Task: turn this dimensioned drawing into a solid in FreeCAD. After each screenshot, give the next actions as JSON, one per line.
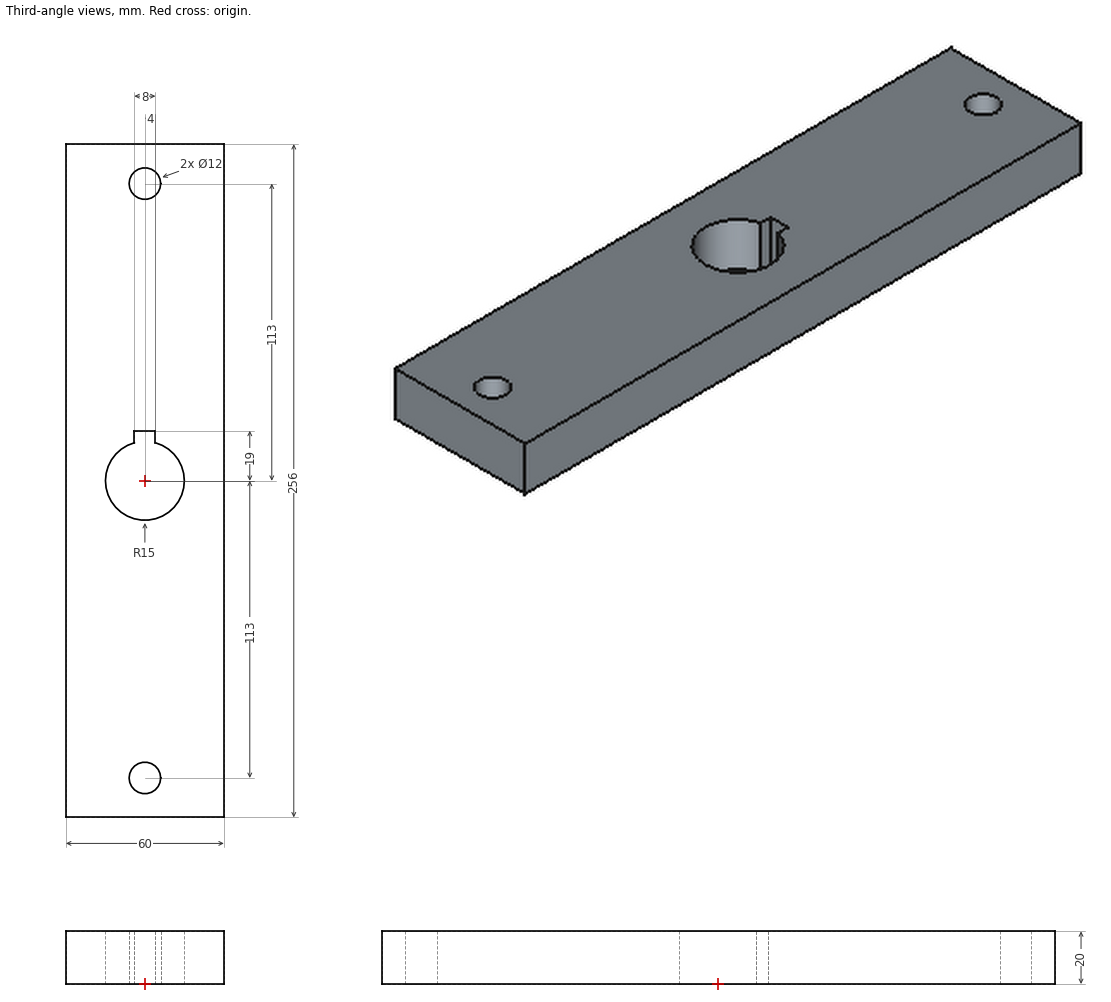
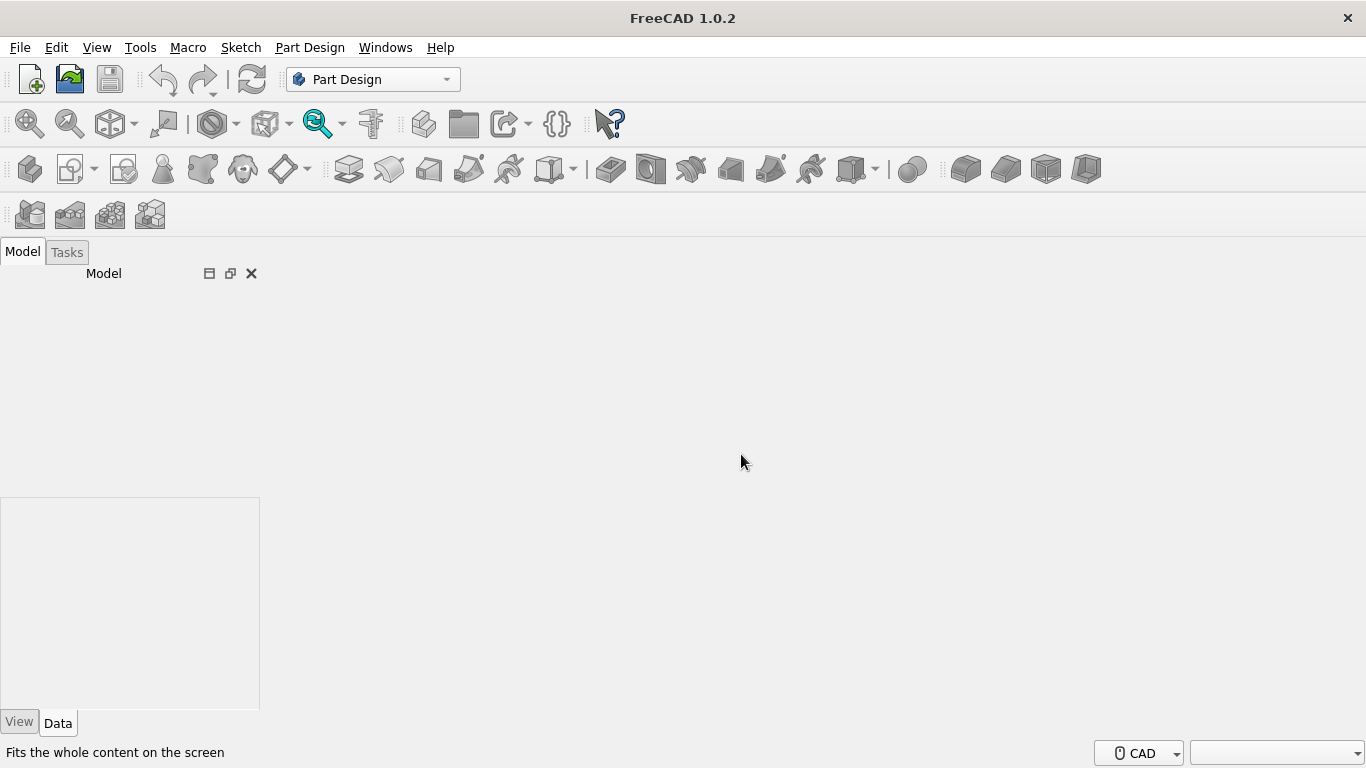
{"action": "key", "text": "ctrl+n"}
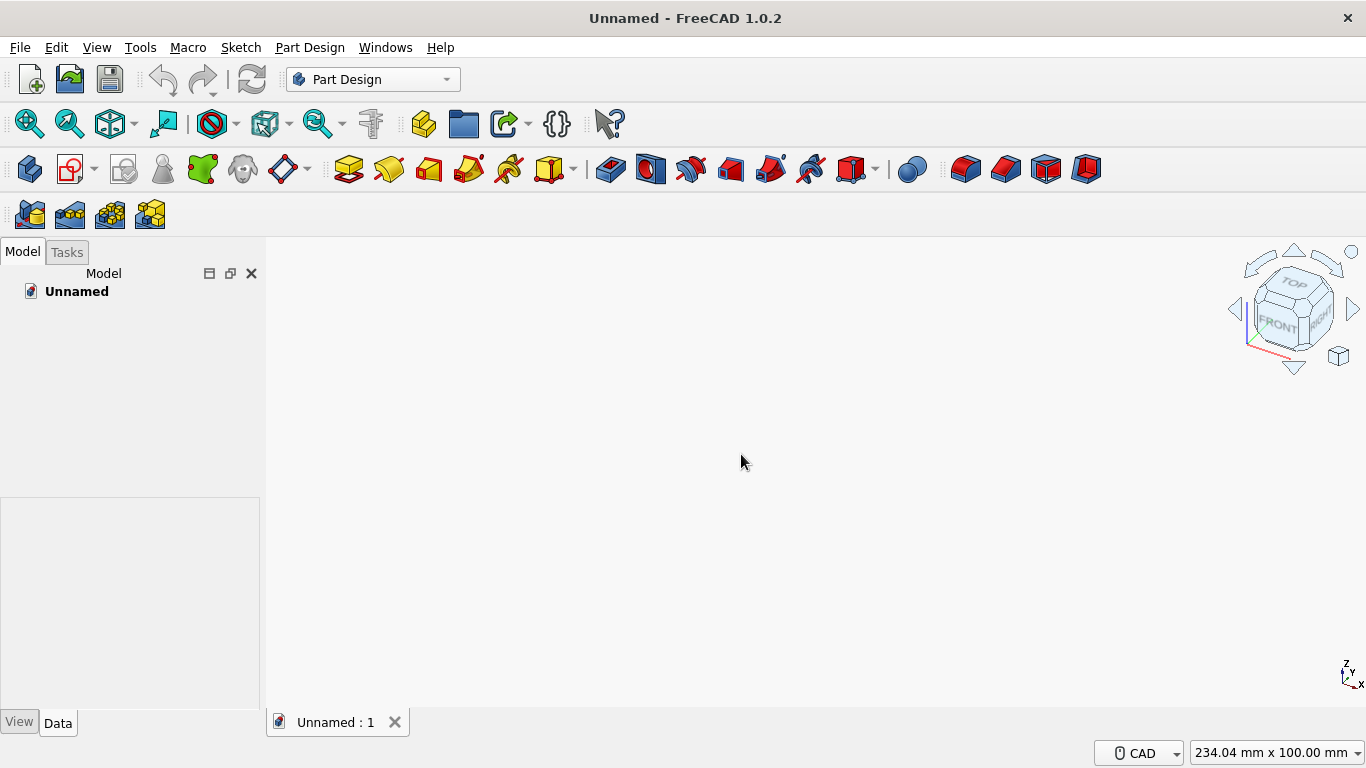
{"action": "left_click", "coordinate": [70, 170]}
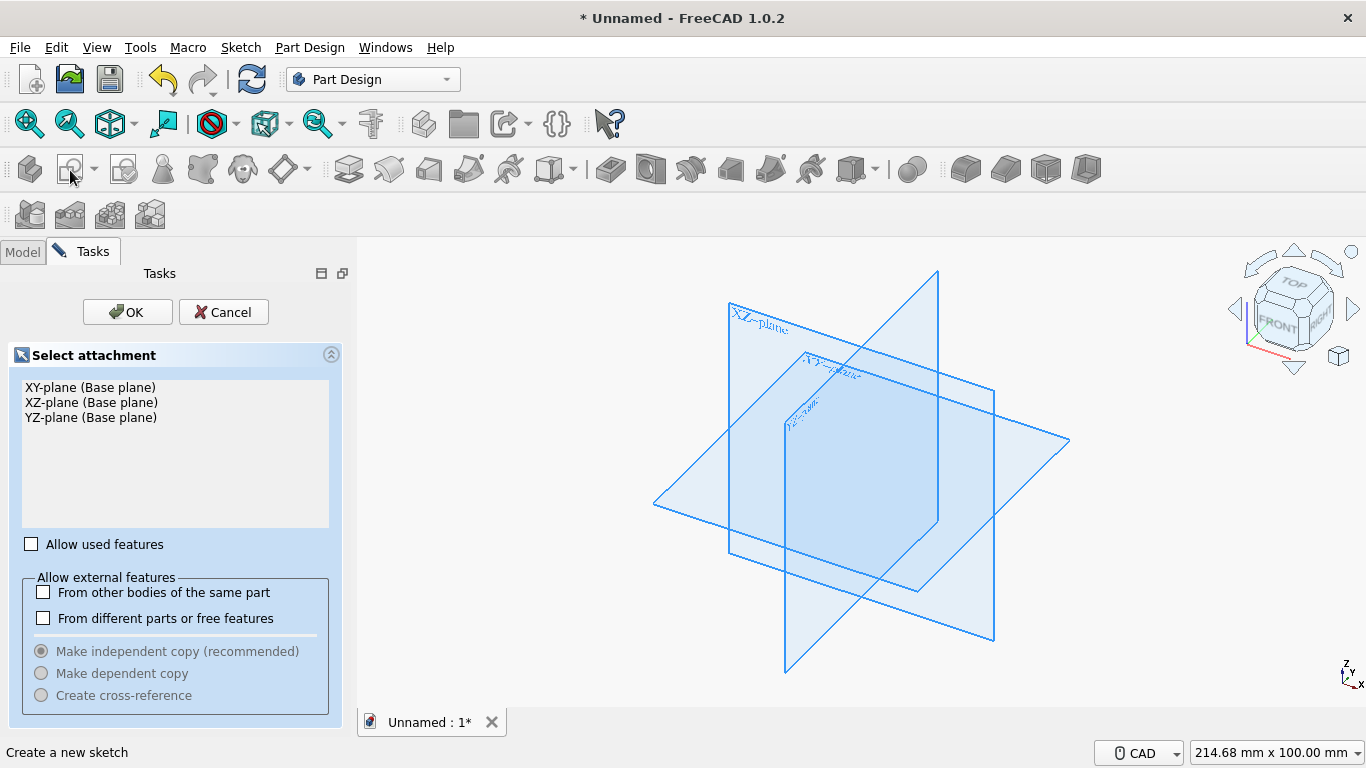
{"action": "left_click", "coordinate": [82, 388]}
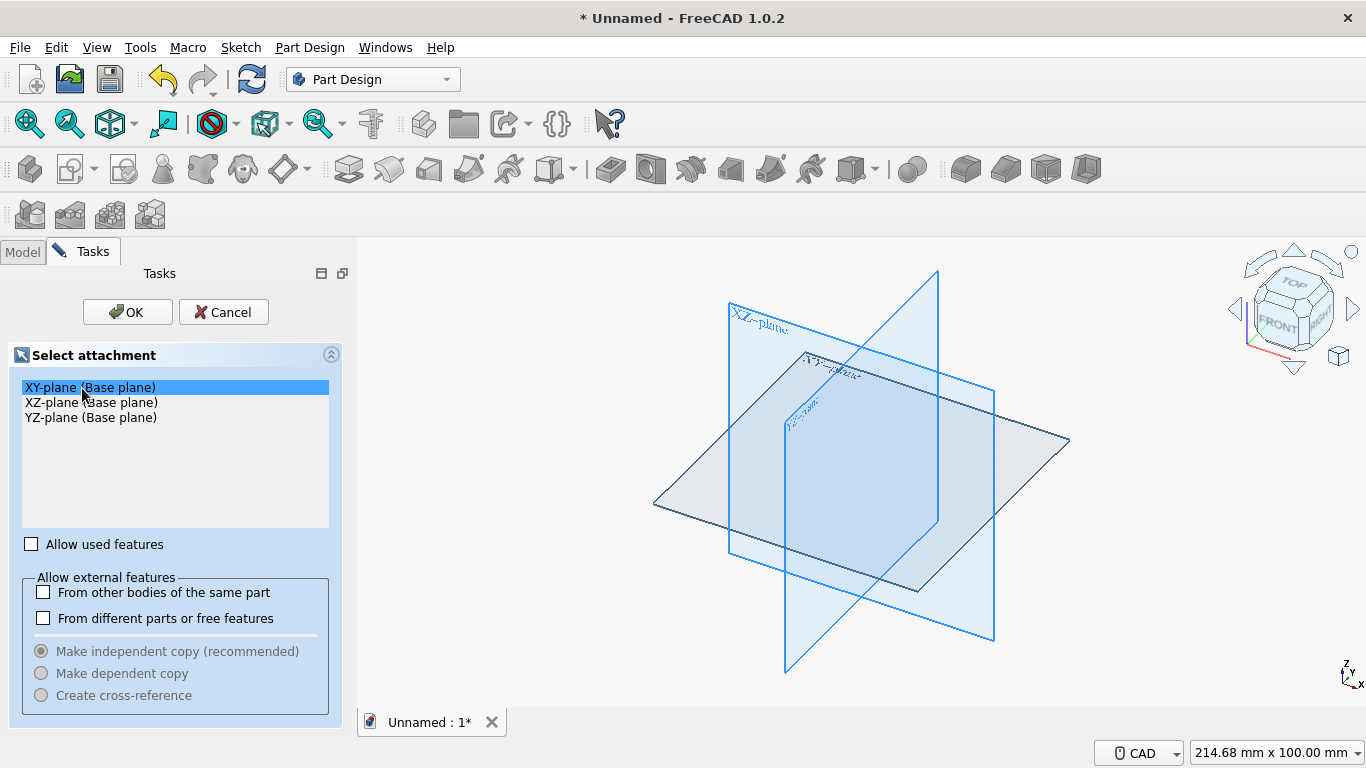
{"action": "left_click", "coordinate": [128, 312]}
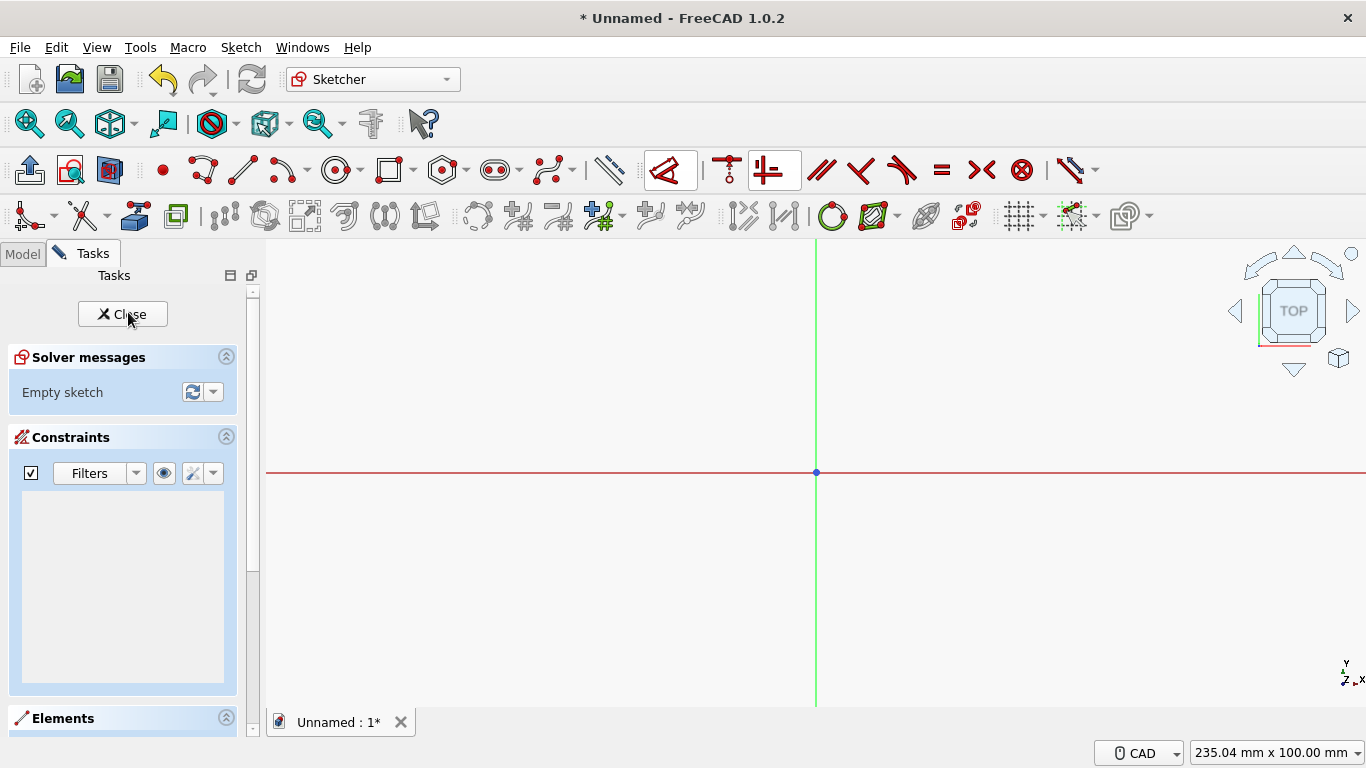
{"action": "scroll", "coordinate": [725, 473], "scroll_direction": "down", "scroll_amount": 7}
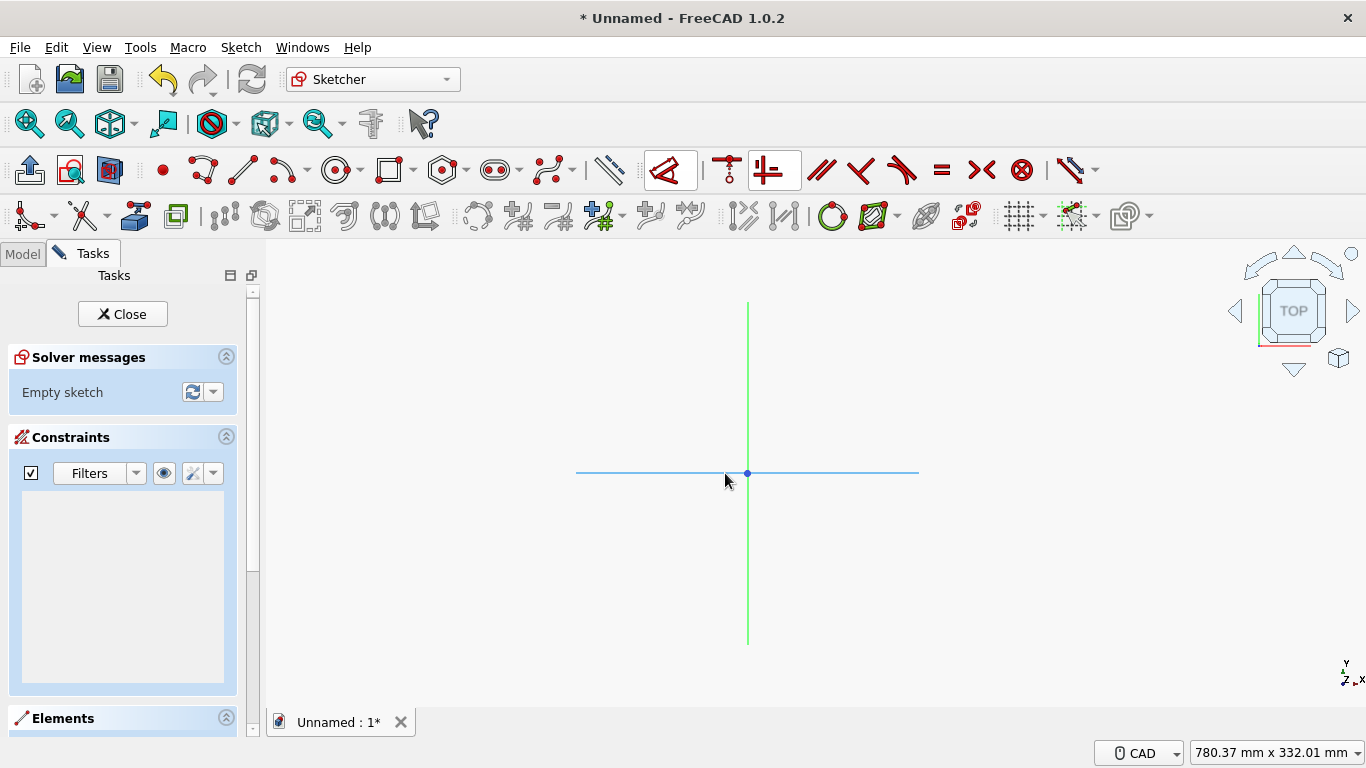
{"action": "key", "text": "g v"}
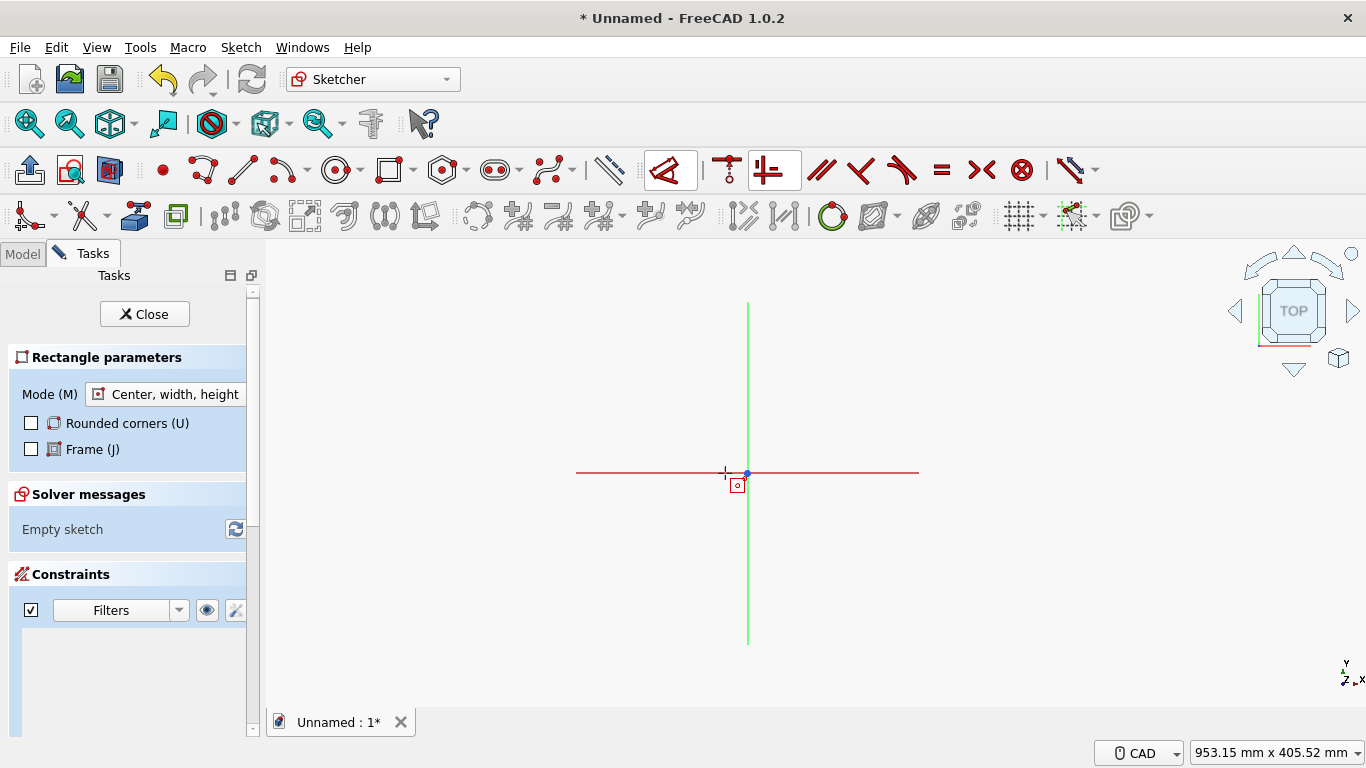
{"action": "left_click", "coordinate": [748, 473]}
{"action": "left_click", "coordinate": [782, 326]}
{"action": "key", "text": "Escape"}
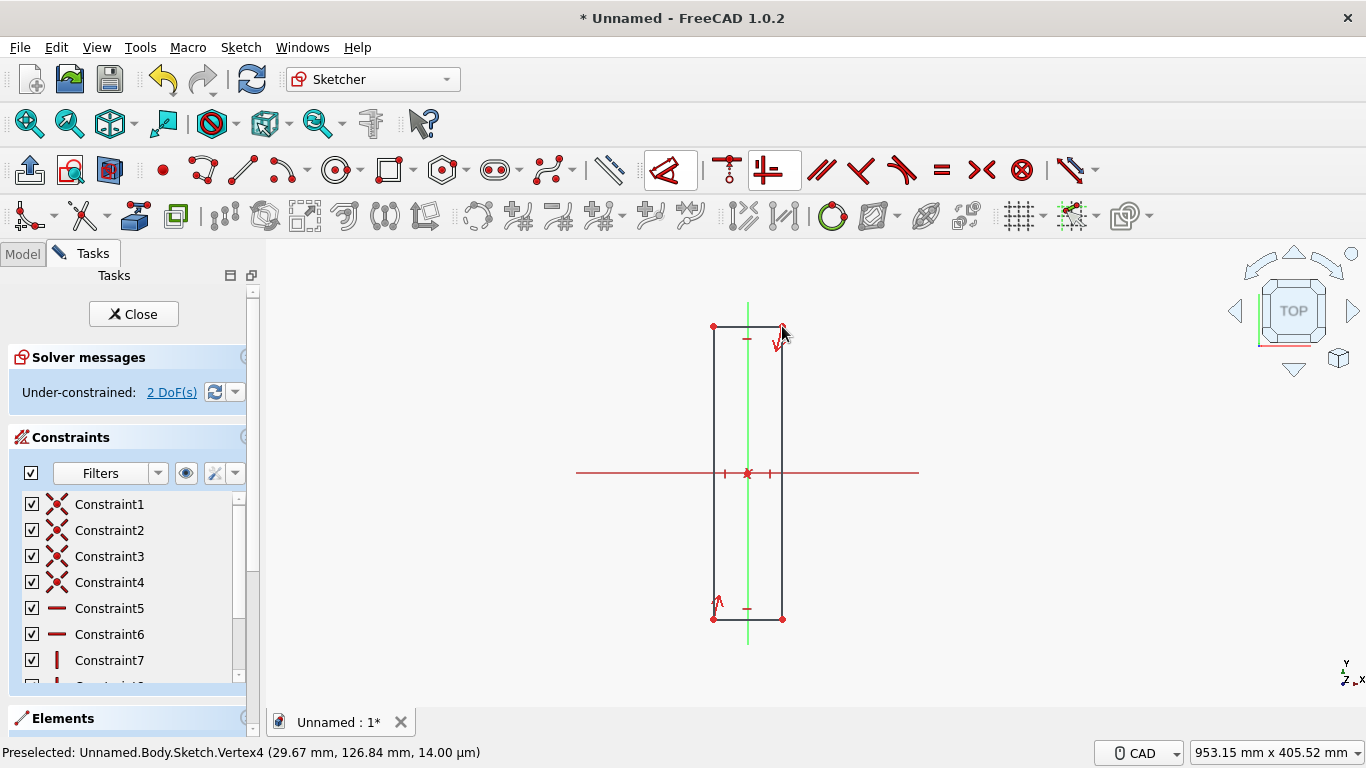
{"action": "key", "text": "d"}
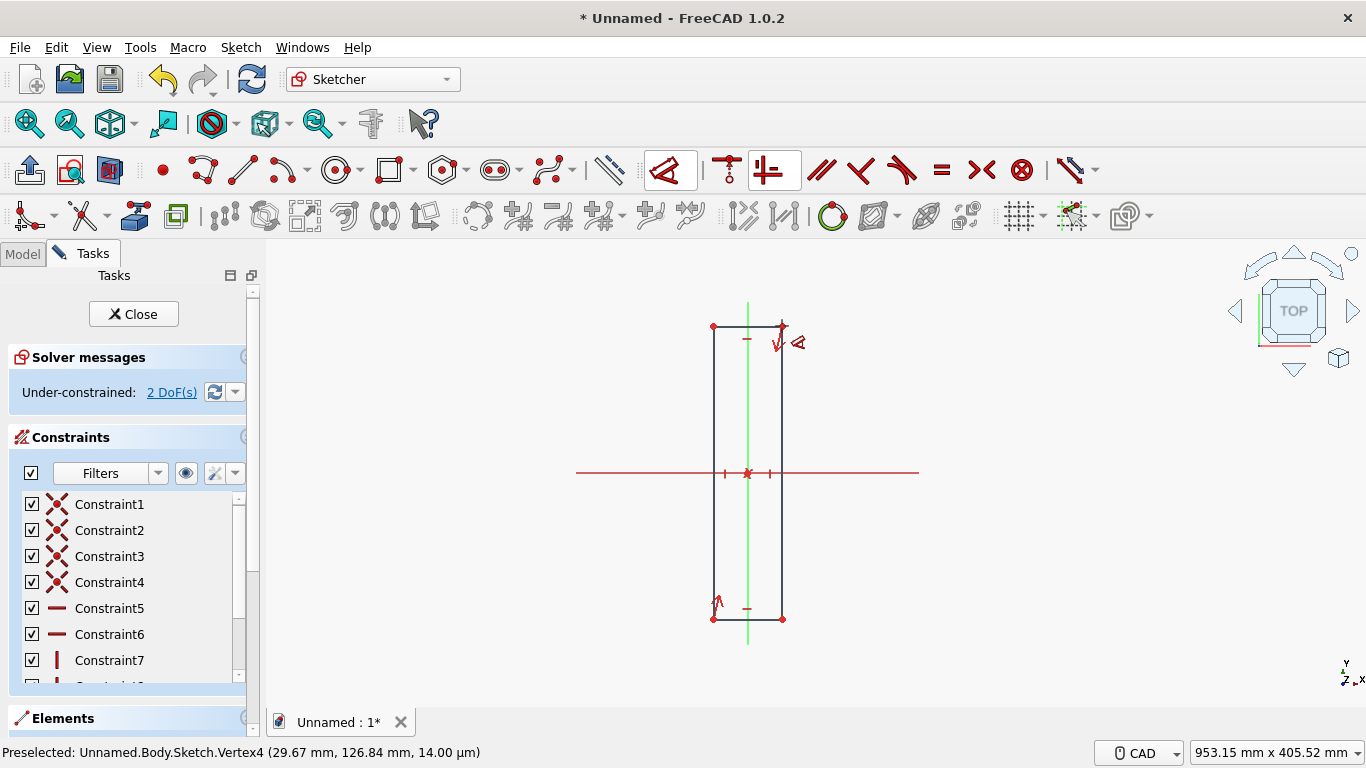
{"action": "left_click", "coordinate": [734, 620]}
{"action": "left_click", "coordinate": [732, 654]}